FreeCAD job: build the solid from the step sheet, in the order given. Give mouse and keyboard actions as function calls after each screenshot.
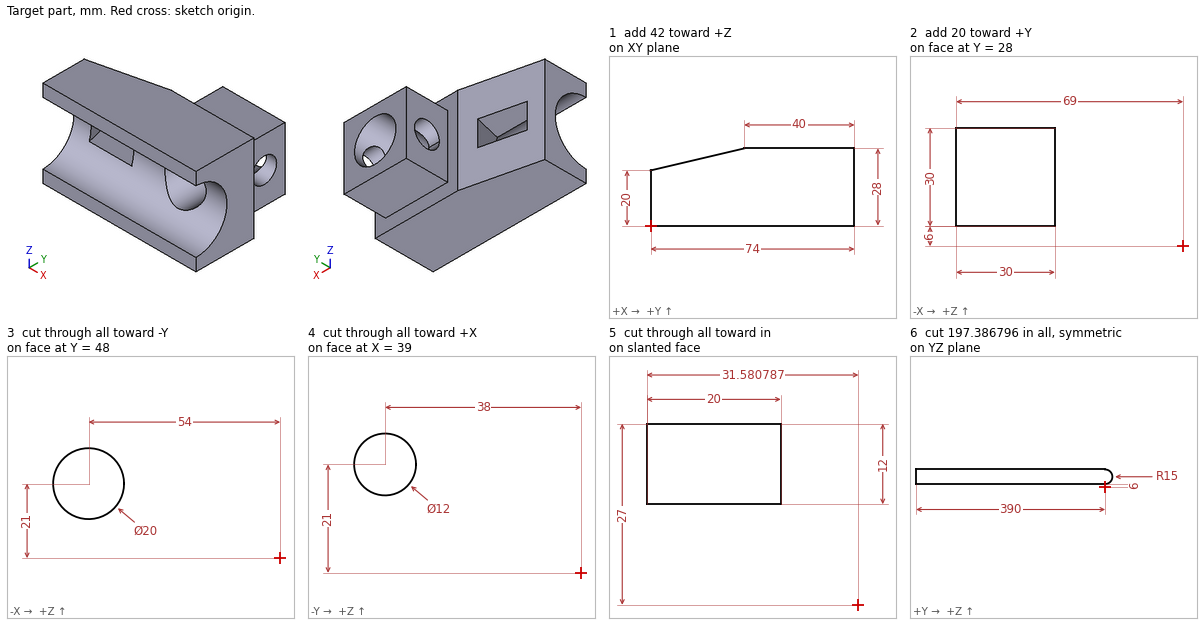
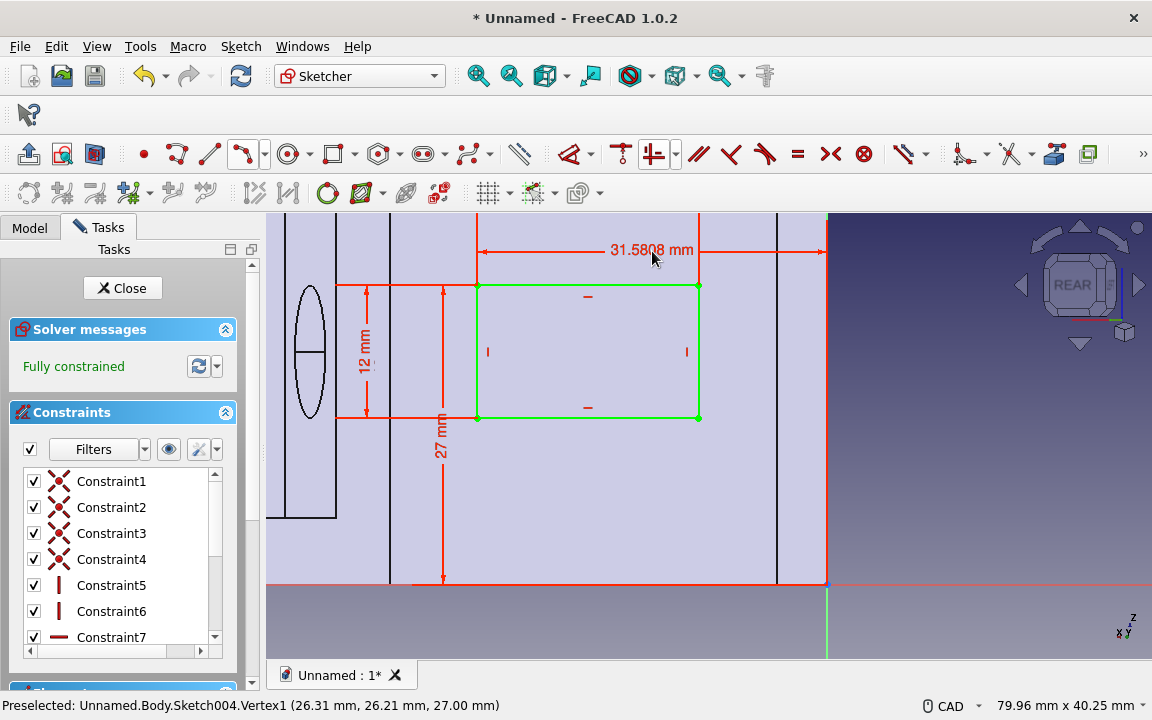
click(123, 288)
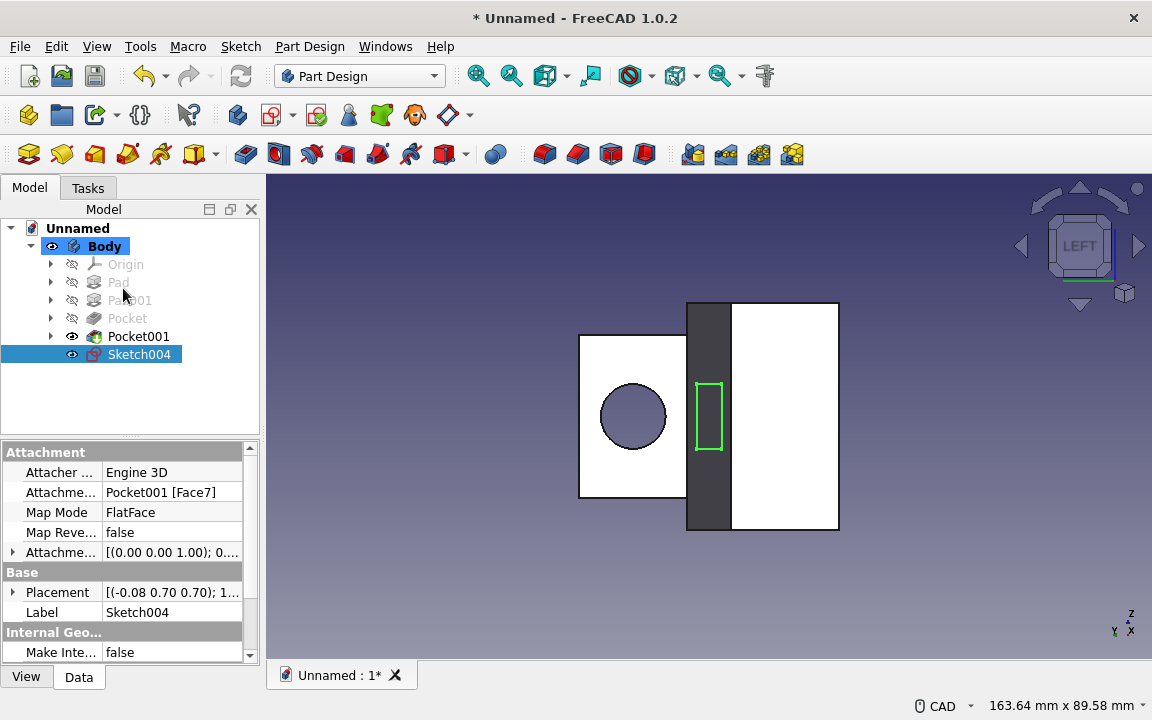
click(246, 154)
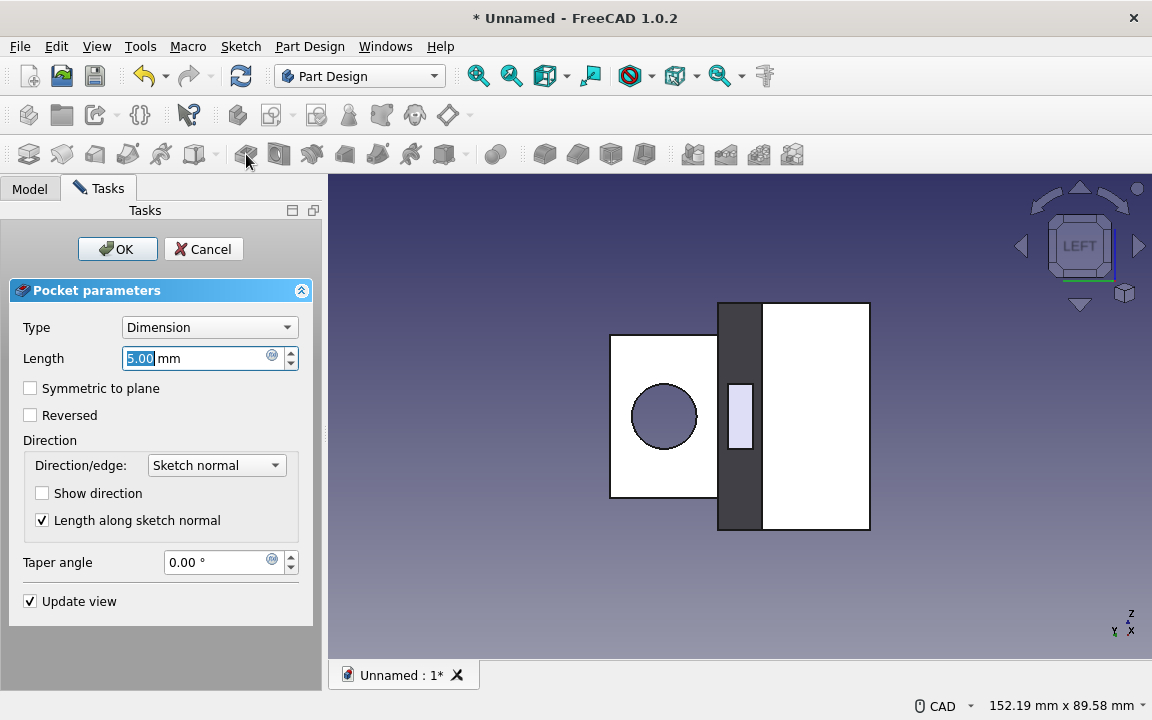
click(210, 328)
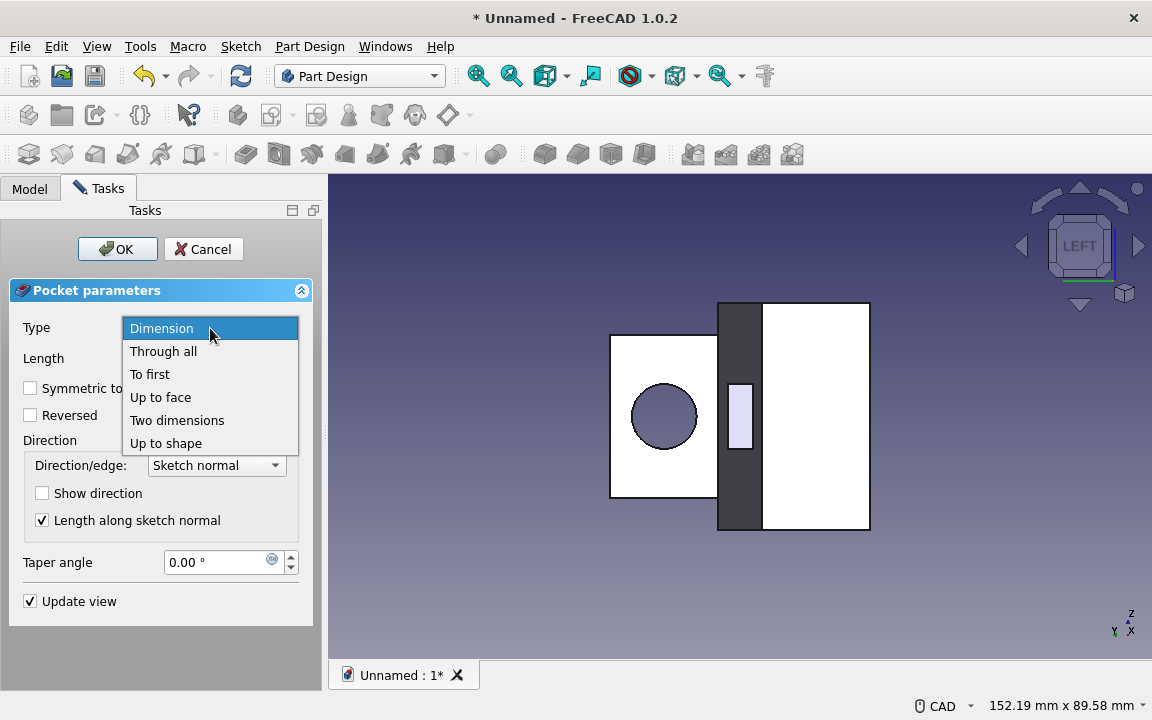
click(208, 352)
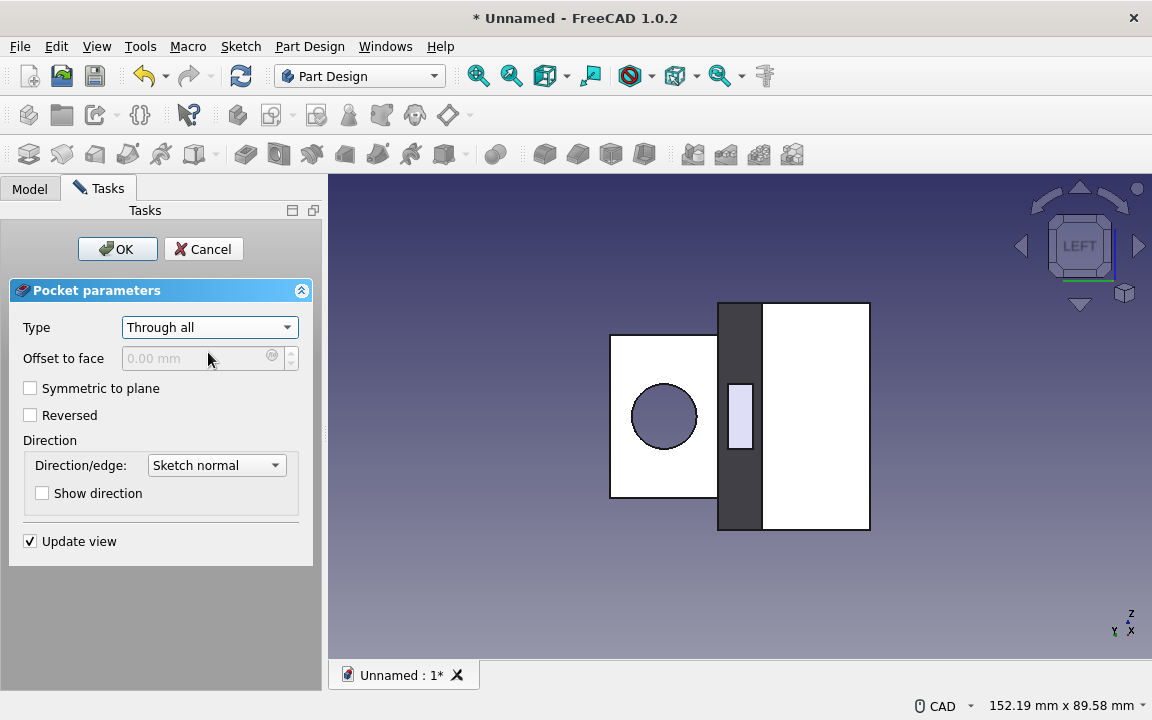
click(118, 249)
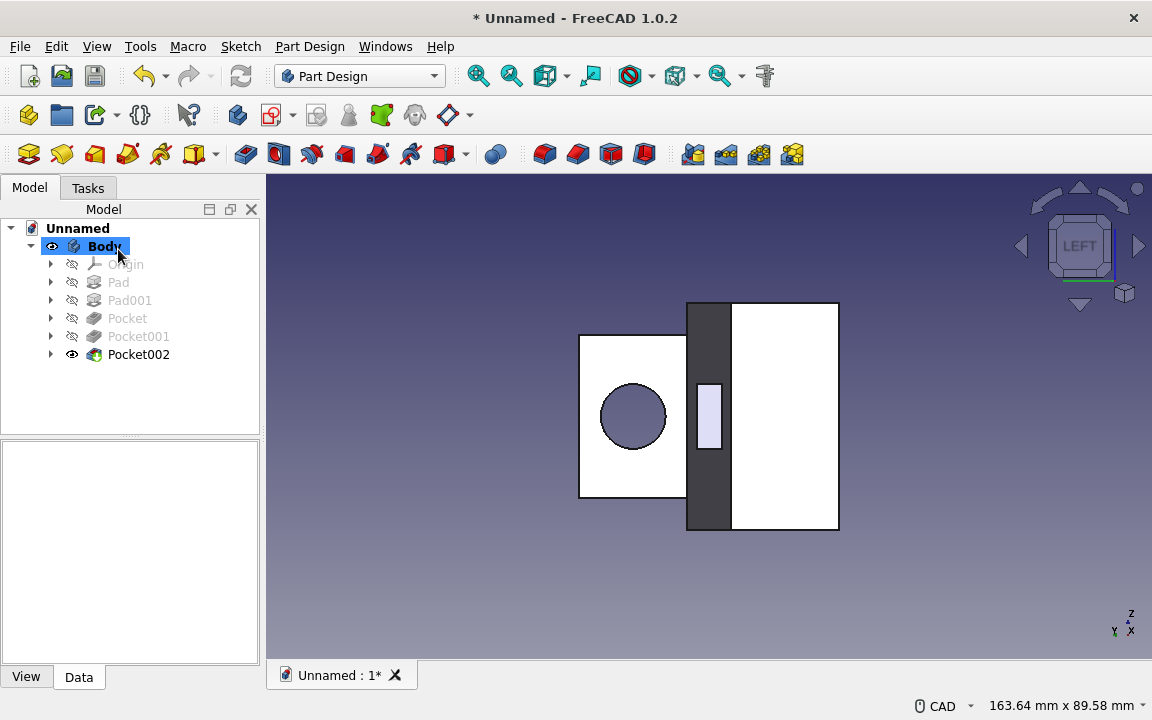
click(270, 116)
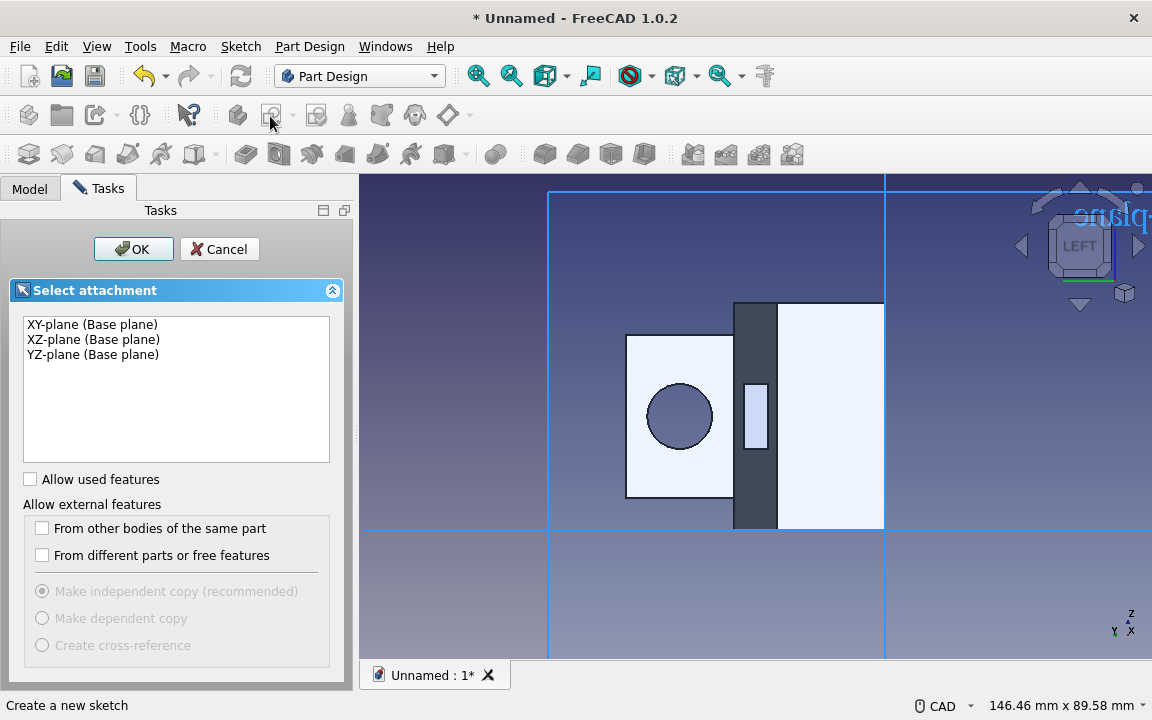
click(84, 354)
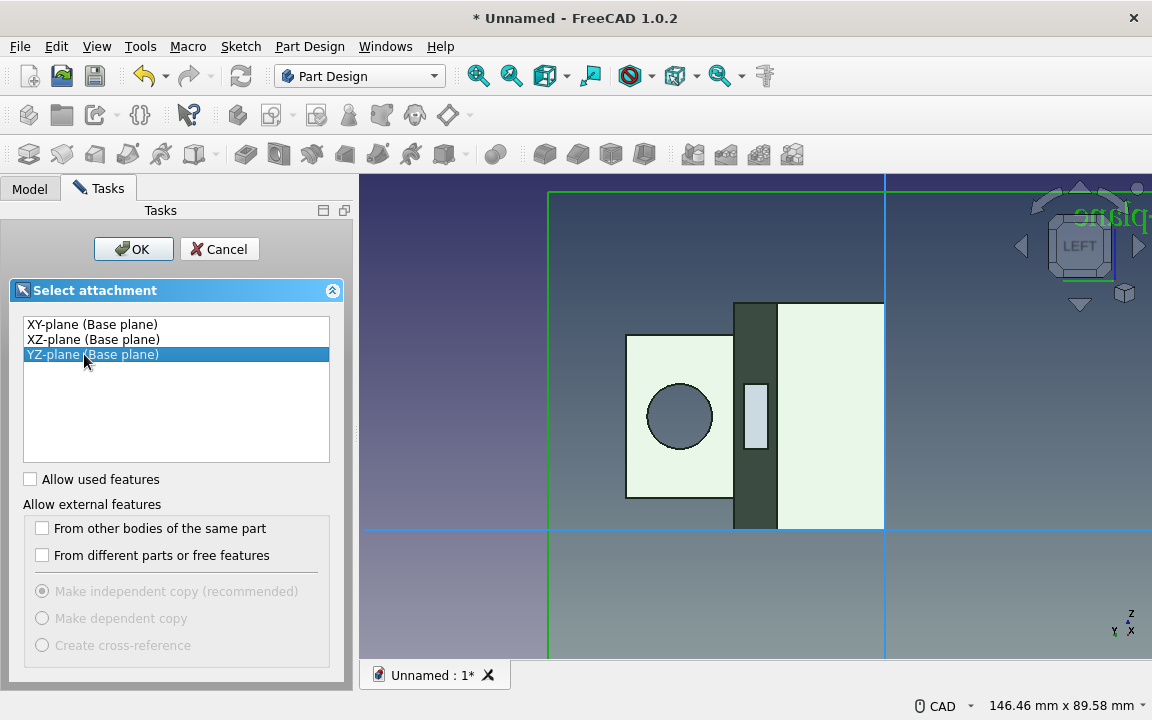
click(134, 249)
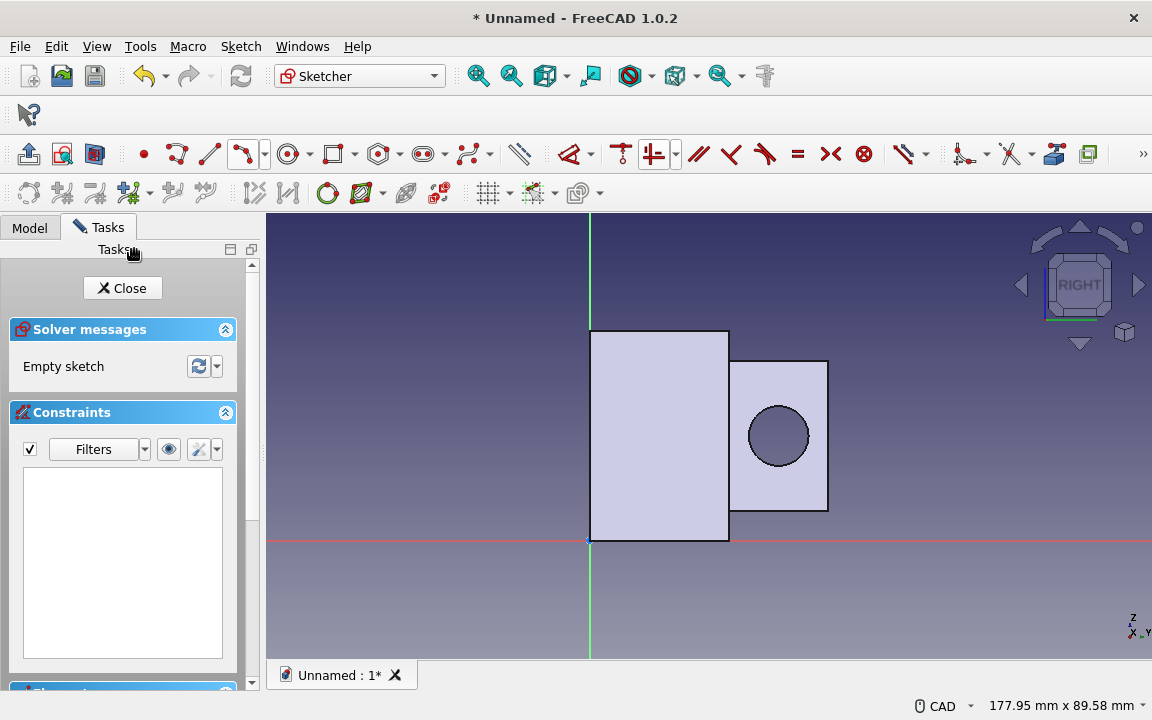
click(95, 154)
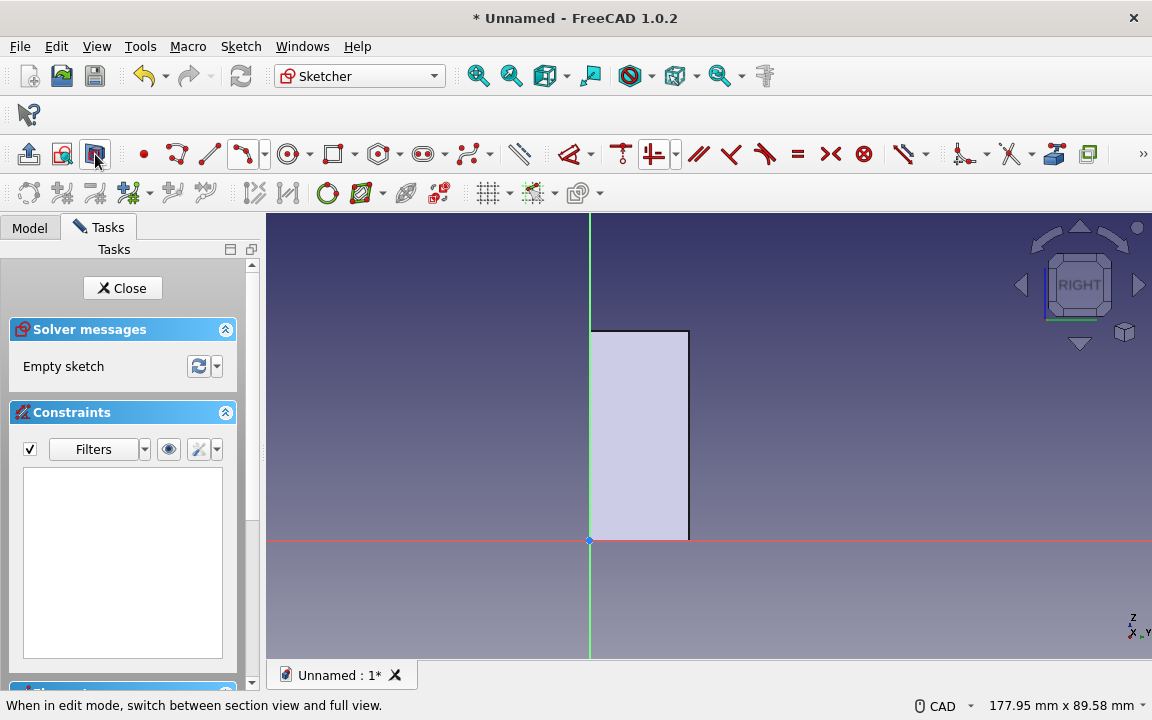
scroll(963, 431, down, 7)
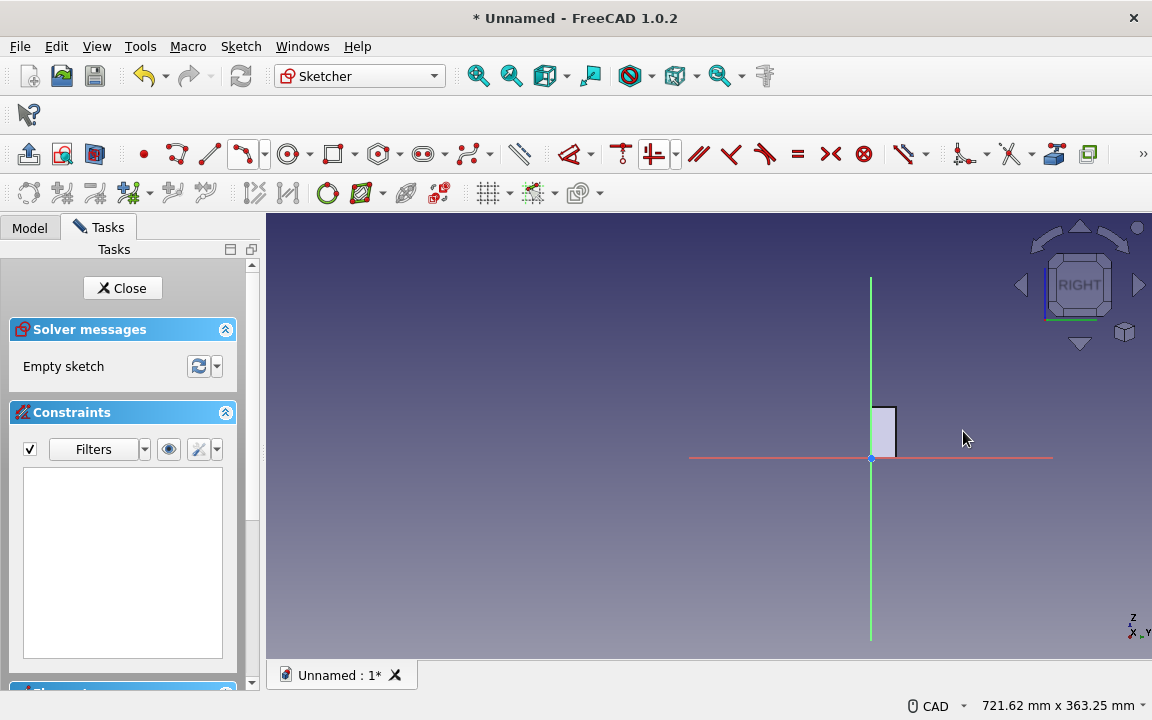
click(177, 154)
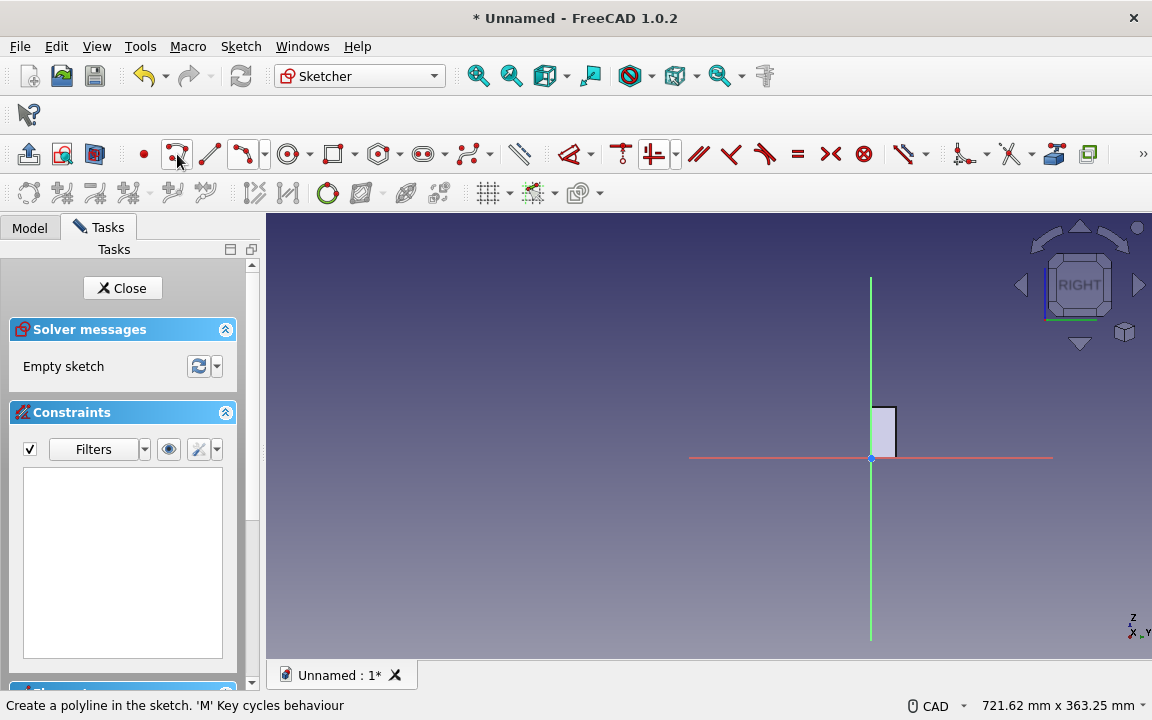
scroll(871, 451, up, 4)